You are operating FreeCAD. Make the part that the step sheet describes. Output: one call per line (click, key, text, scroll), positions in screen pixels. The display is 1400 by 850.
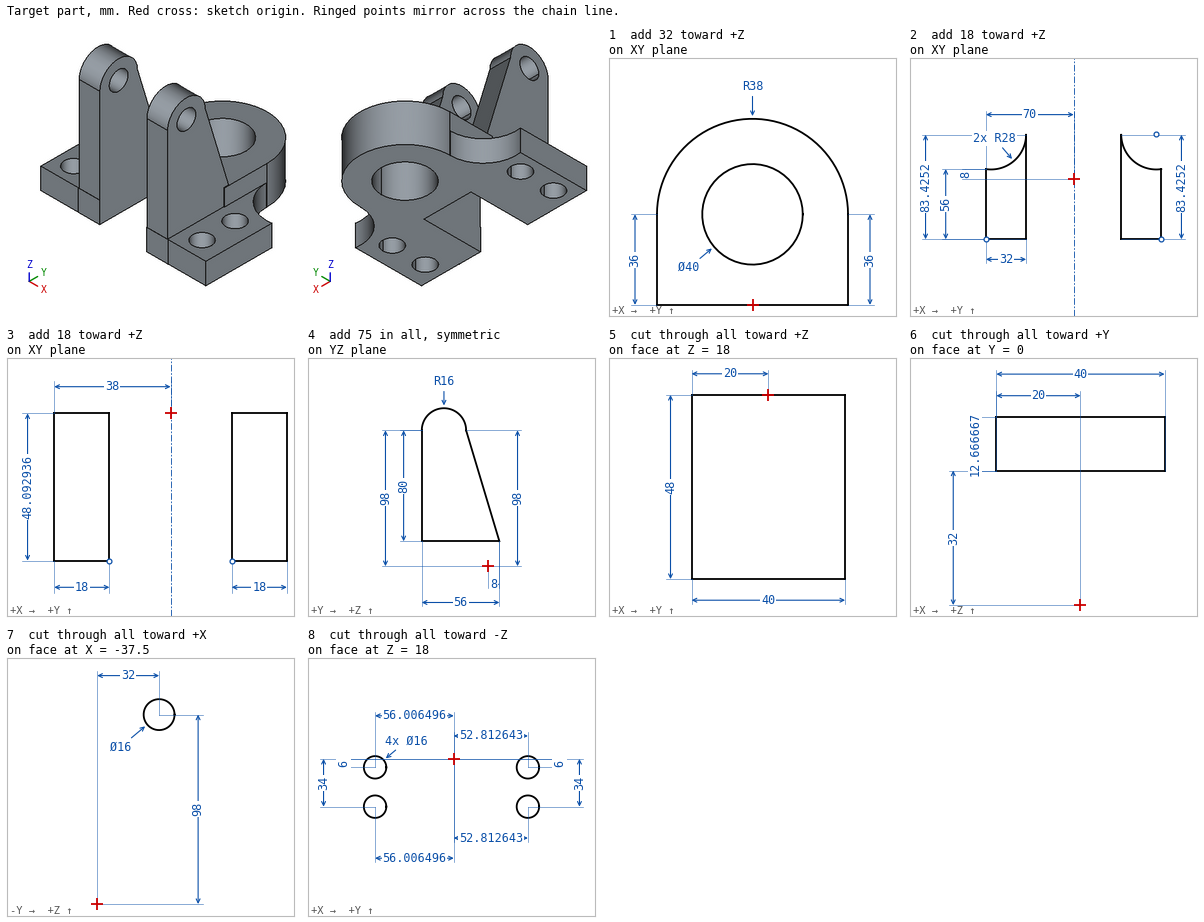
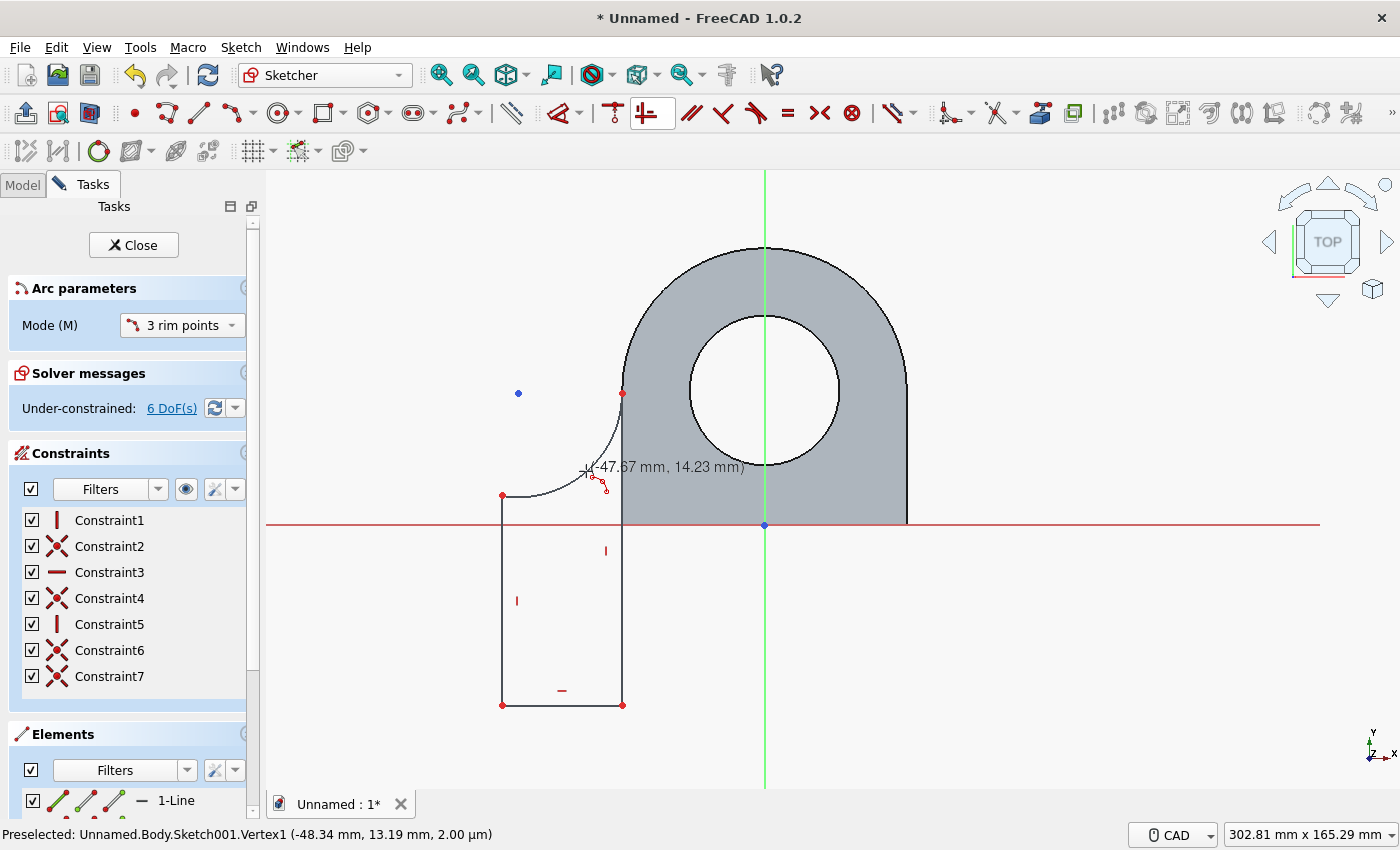
click(168, 114)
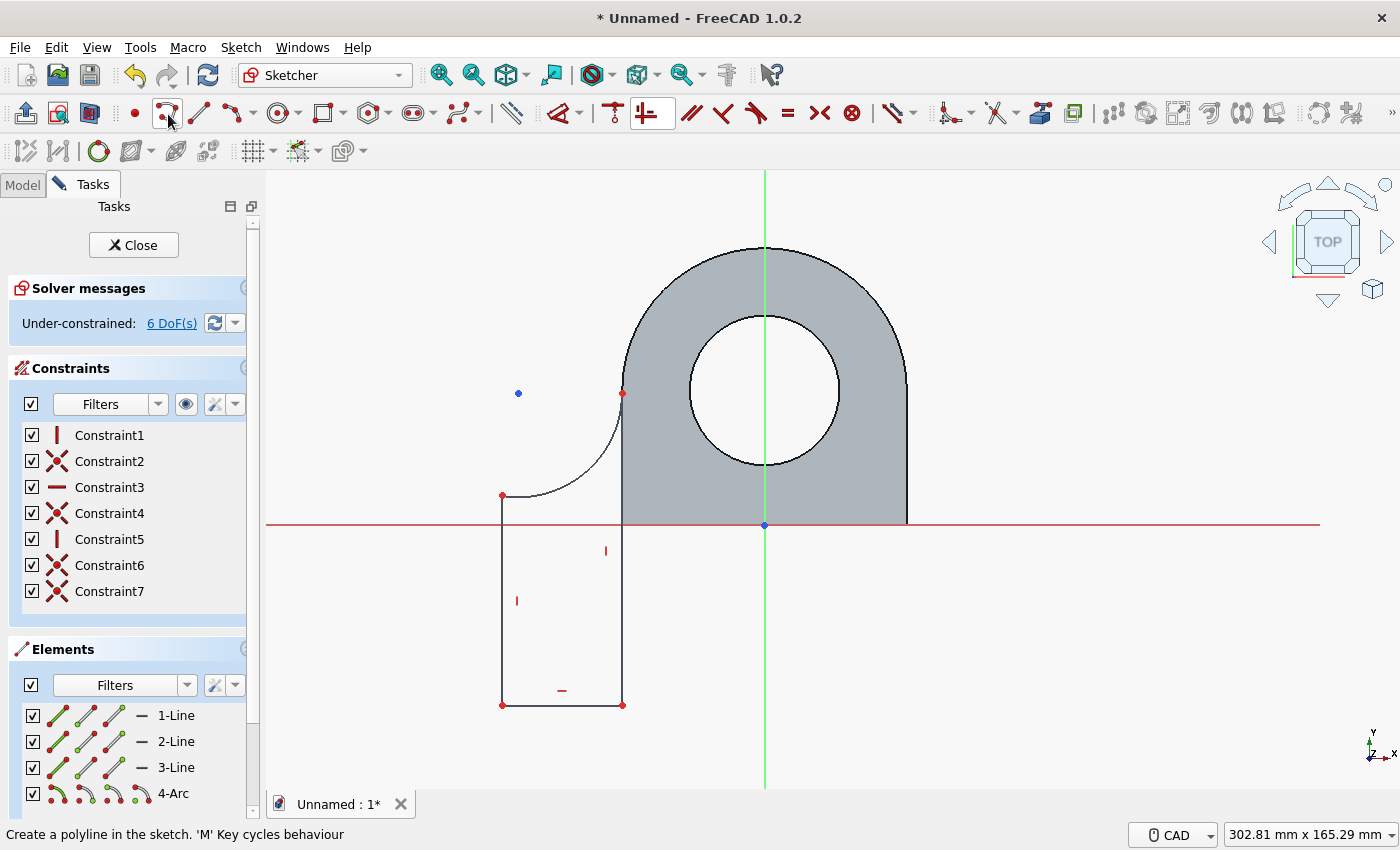
click(907, 393)
click(907, 705)
click(1027, 705)
click(1027, 495)
right_click(1027, 495)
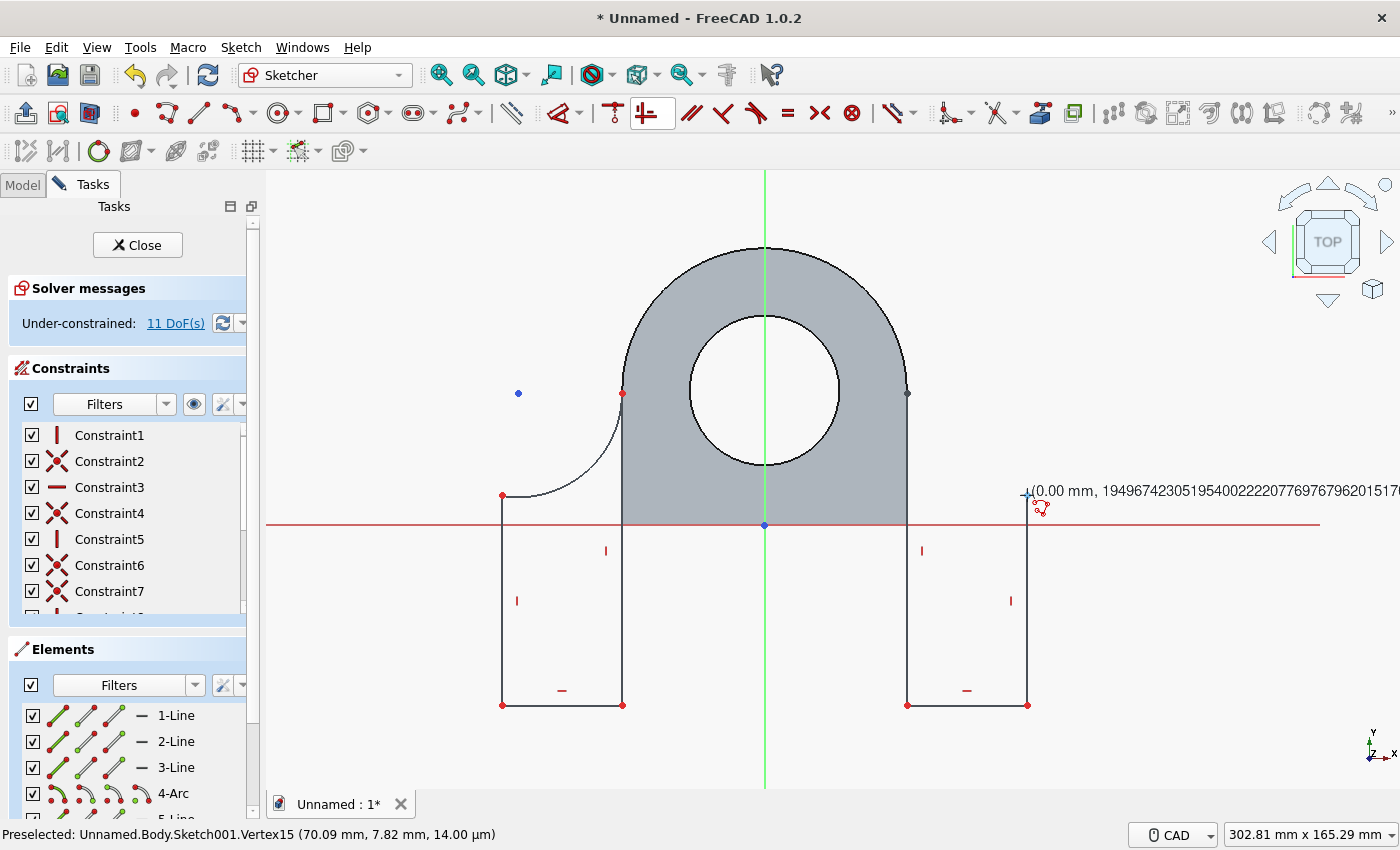
click(232, 114)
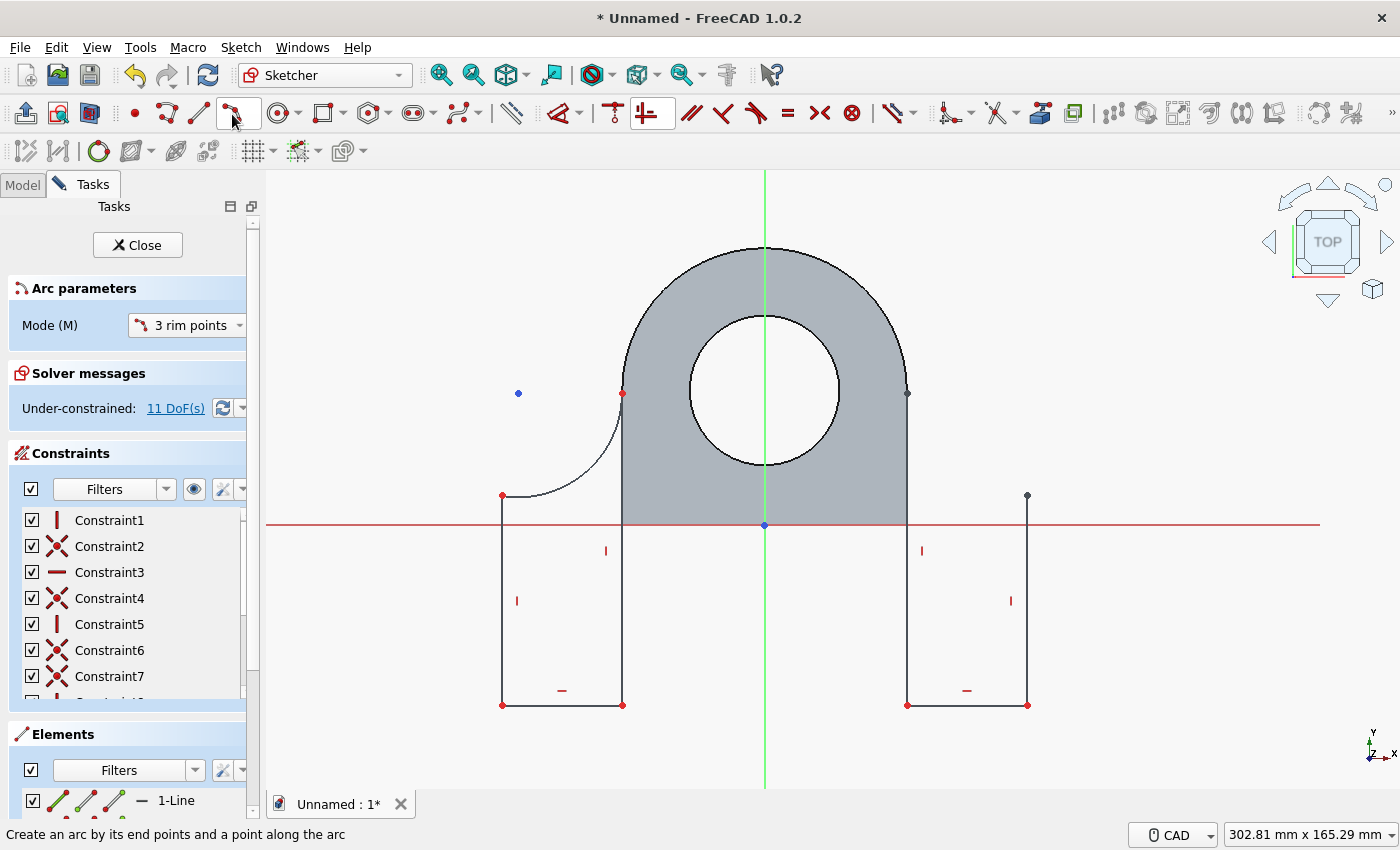
click(1027, 496)
click(907, 394)
click(943, 471)
key(Escape)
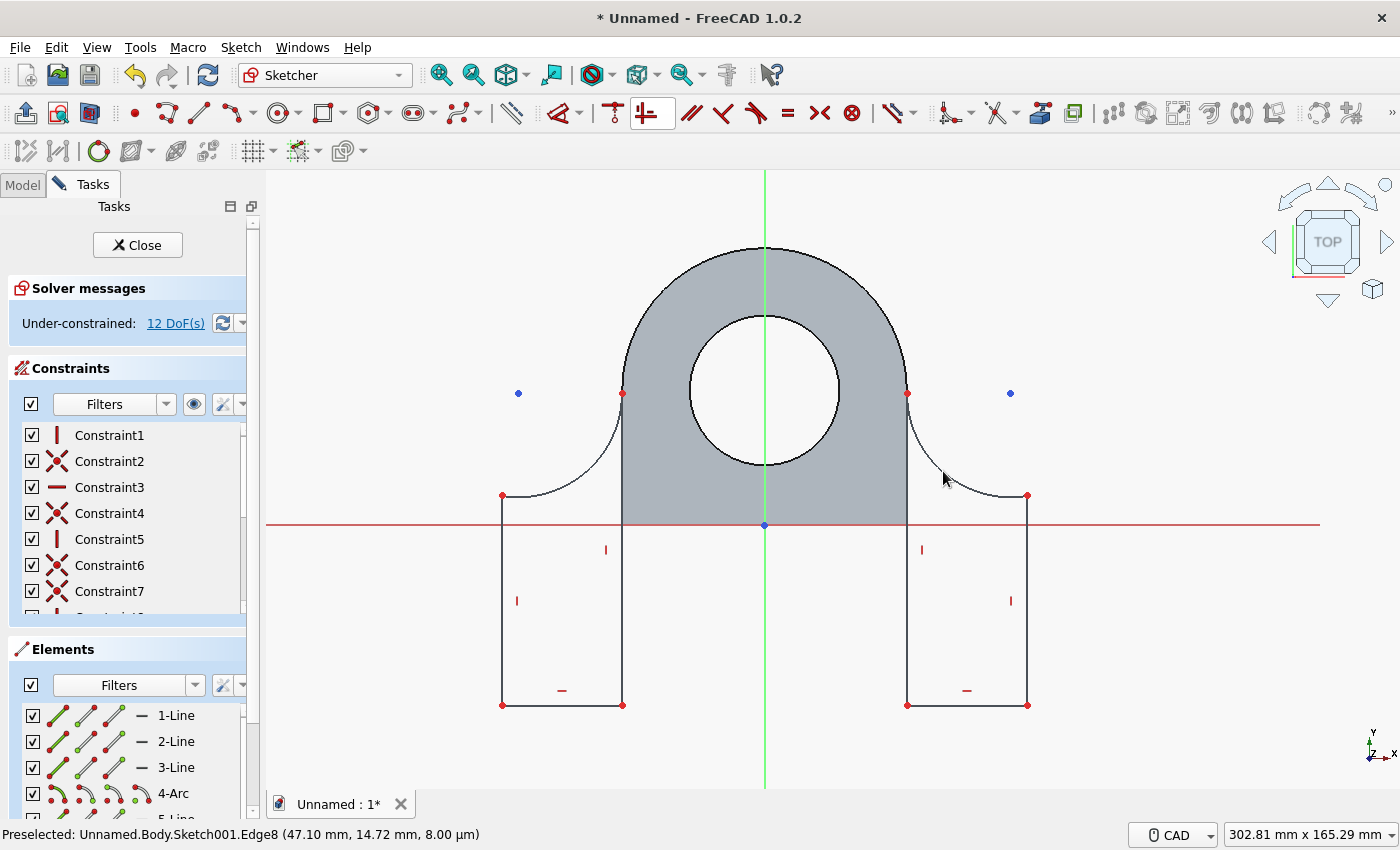
click(555, 491)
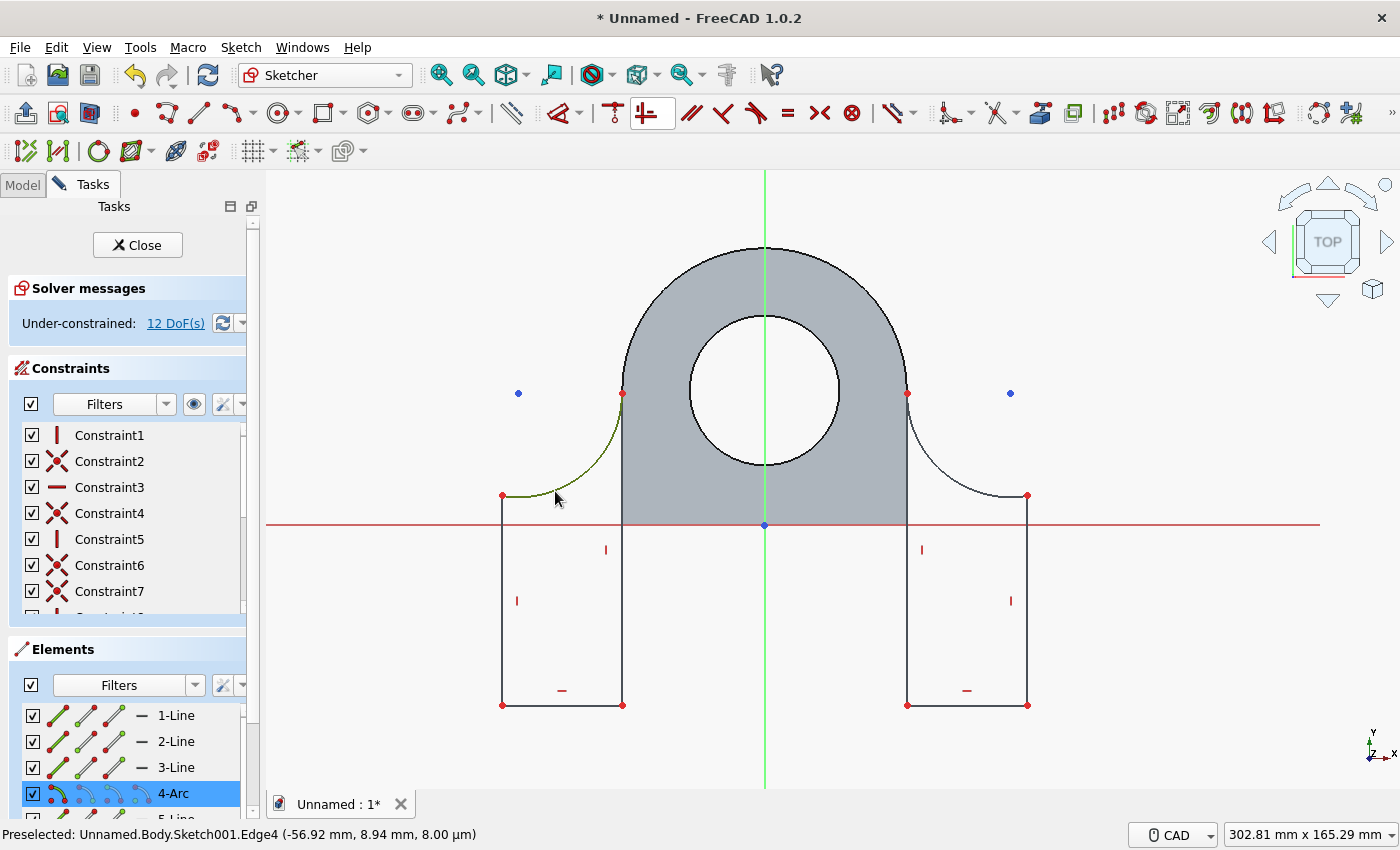
click(921, 445)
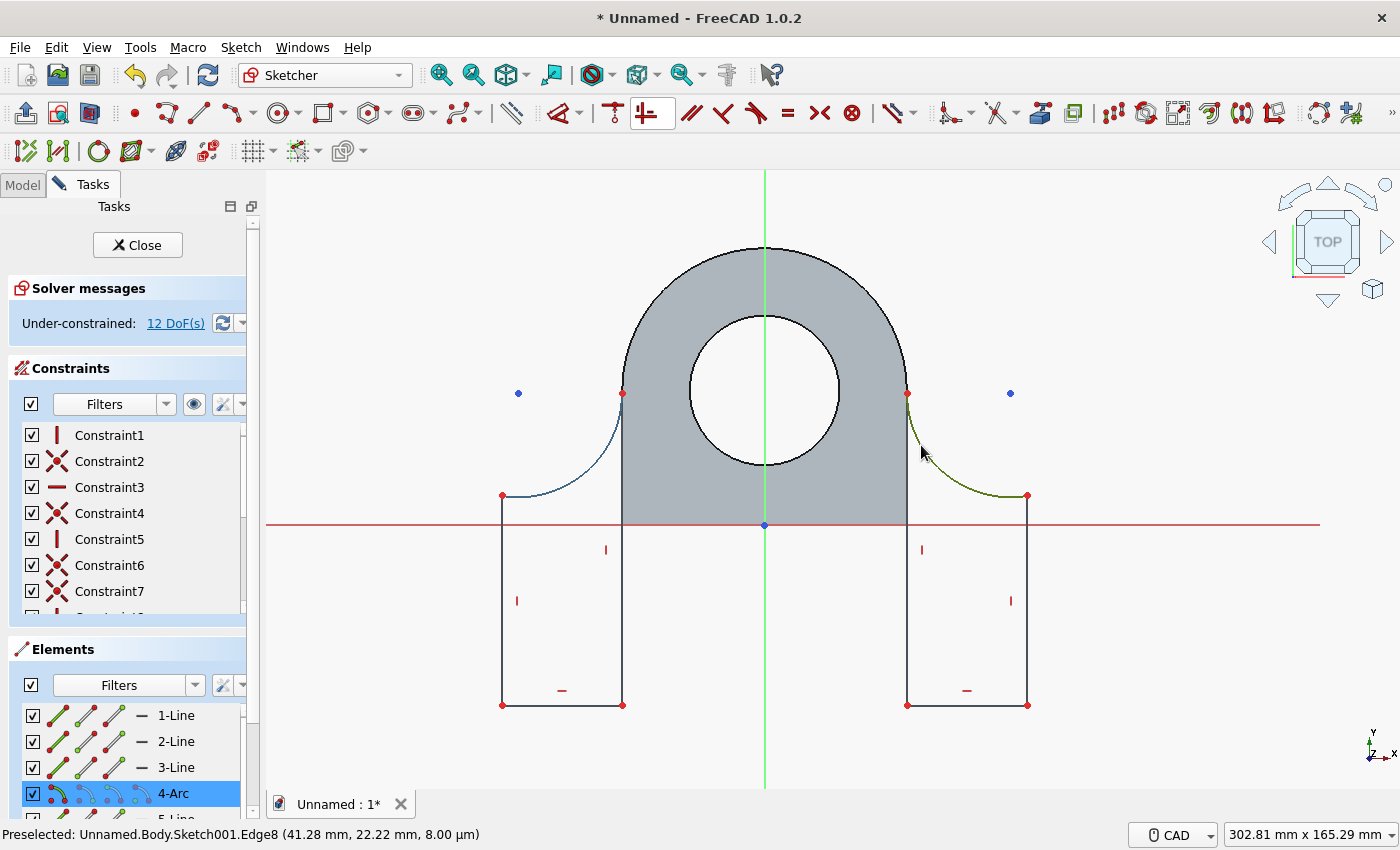
click(788, 114)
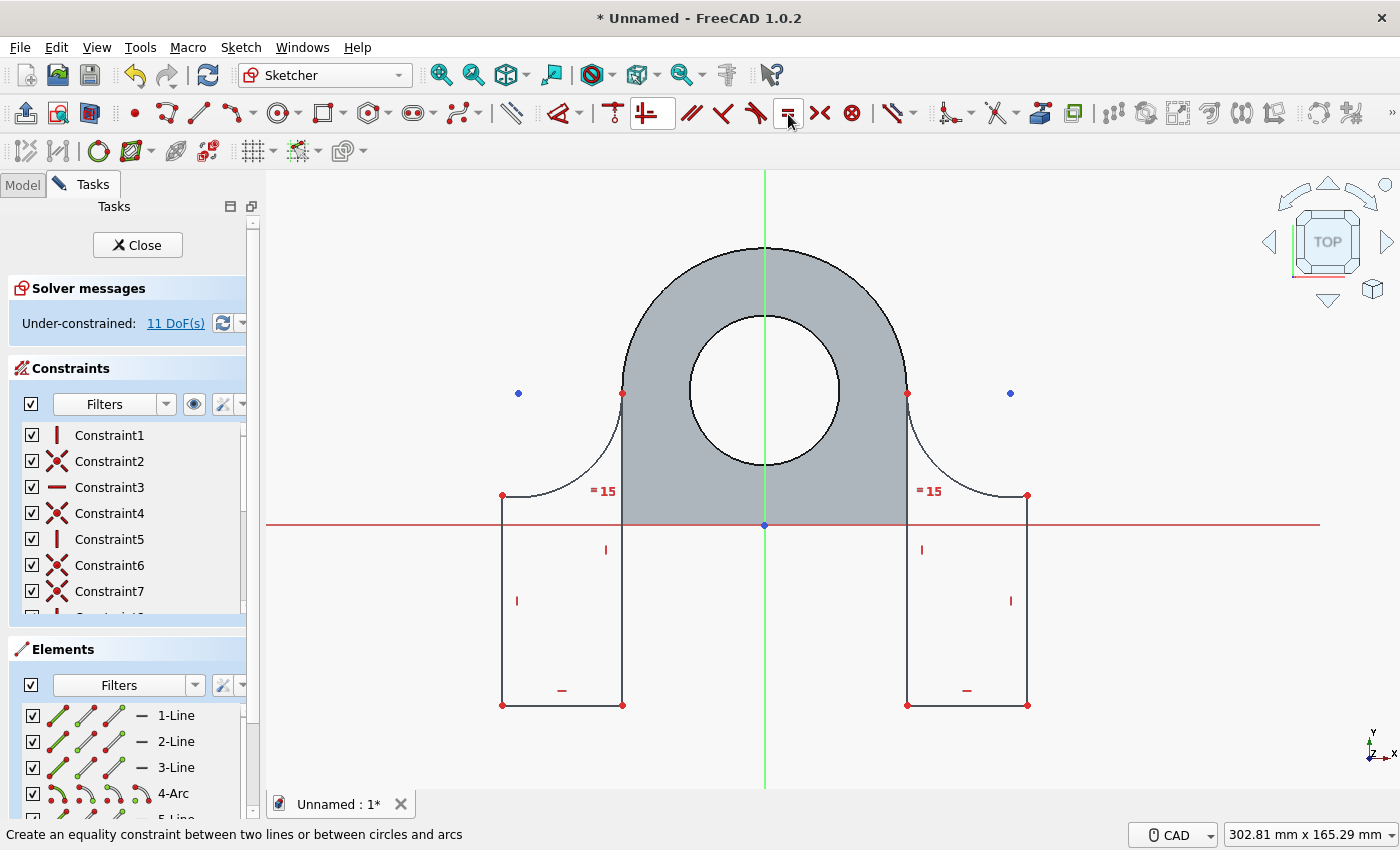
click(518, 393)